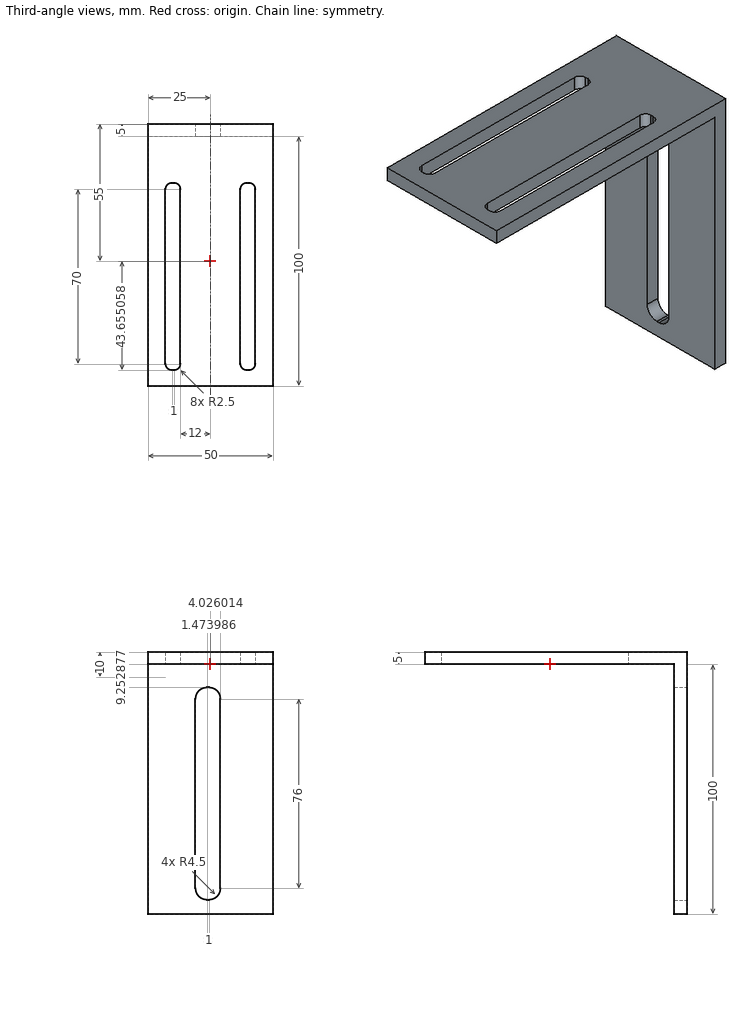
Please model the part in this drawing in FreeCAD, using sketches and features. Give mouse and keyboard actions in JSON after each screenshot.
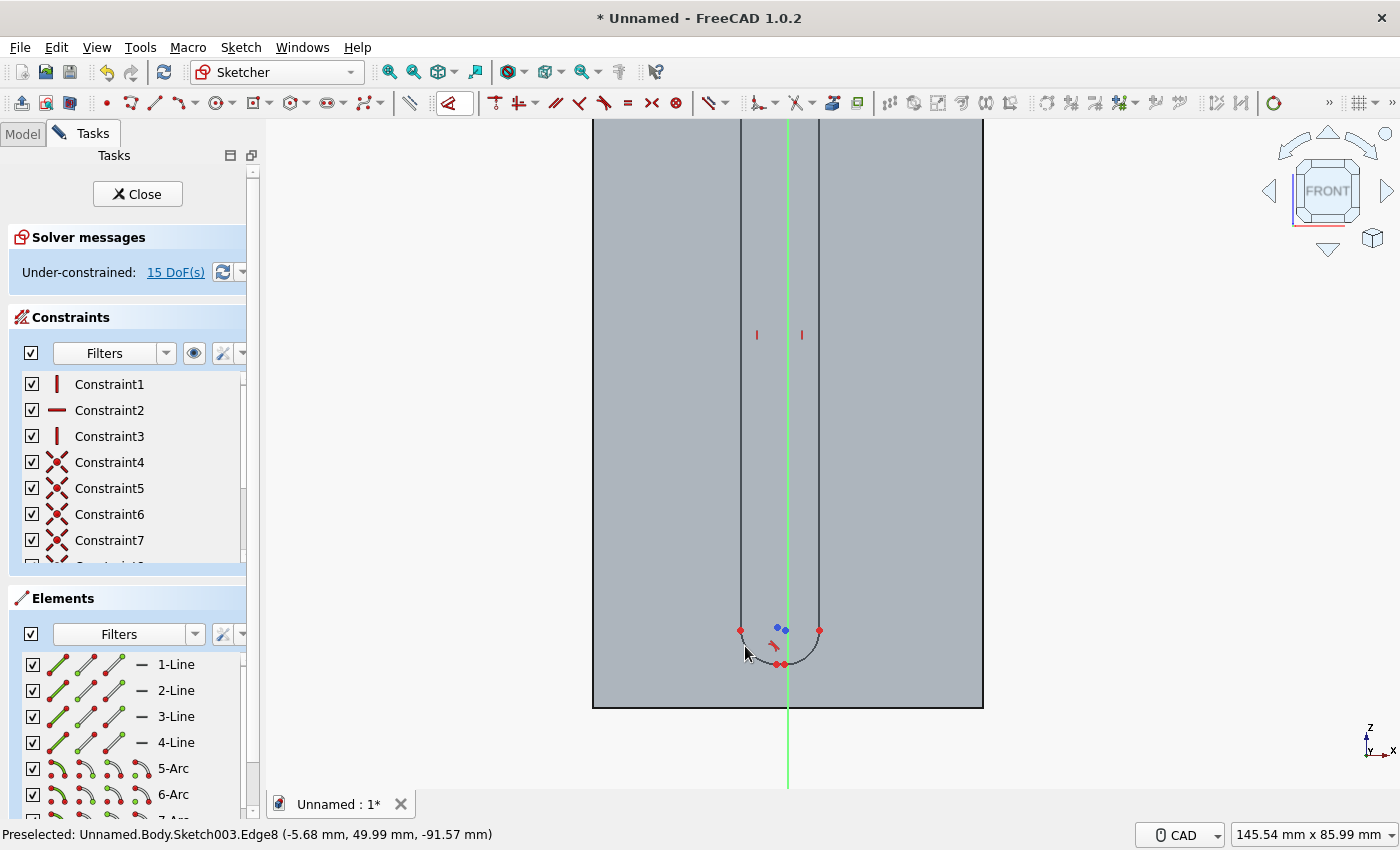
{"action": "left_click", "coordinate": [819, 453]}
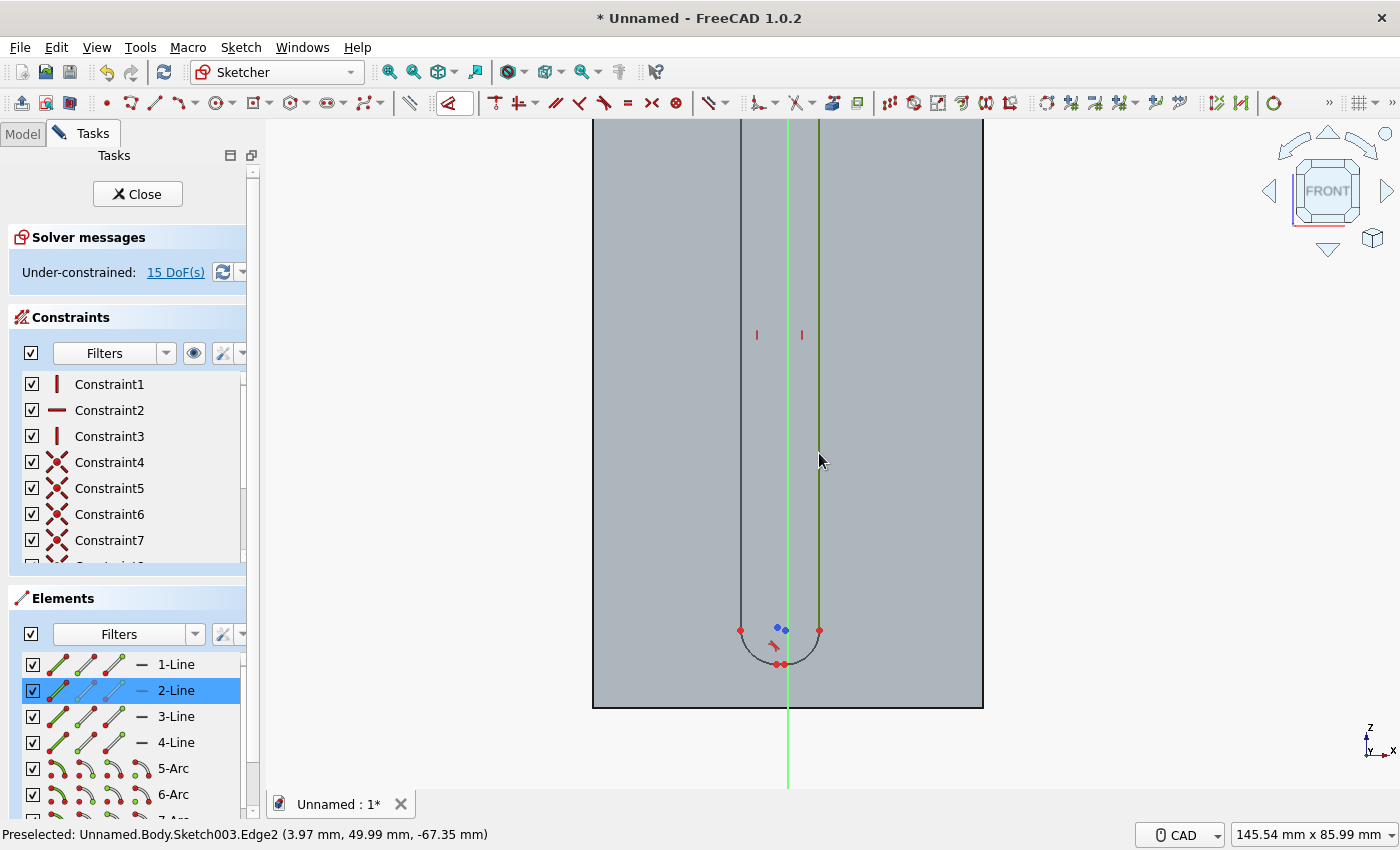
{"action": "left_click", "coordinate": [800, 661]}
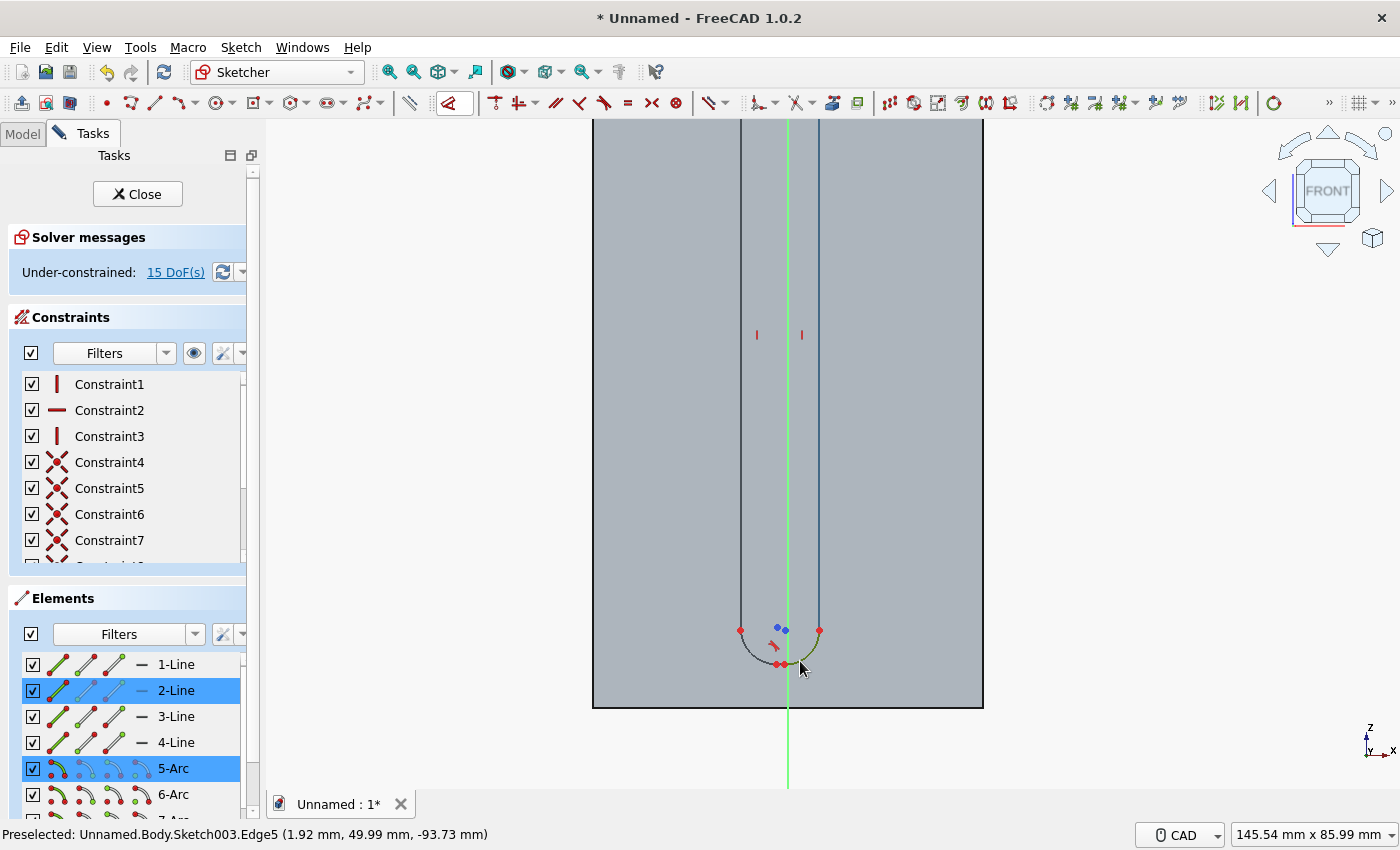
{"action": "left_click", "coordinate": [604, 104]}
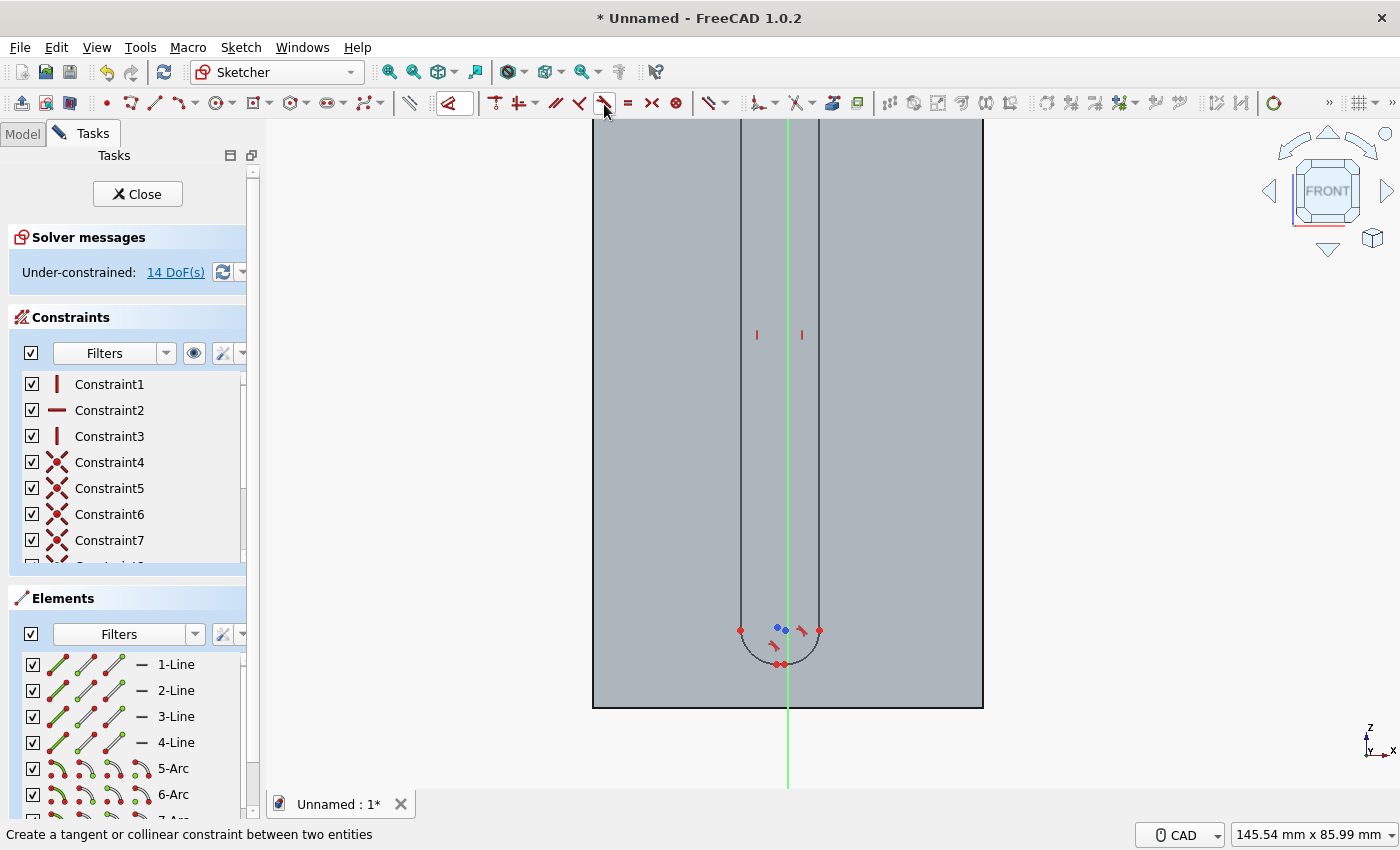
{"action": "left_click", "coordinate": [819, 453]}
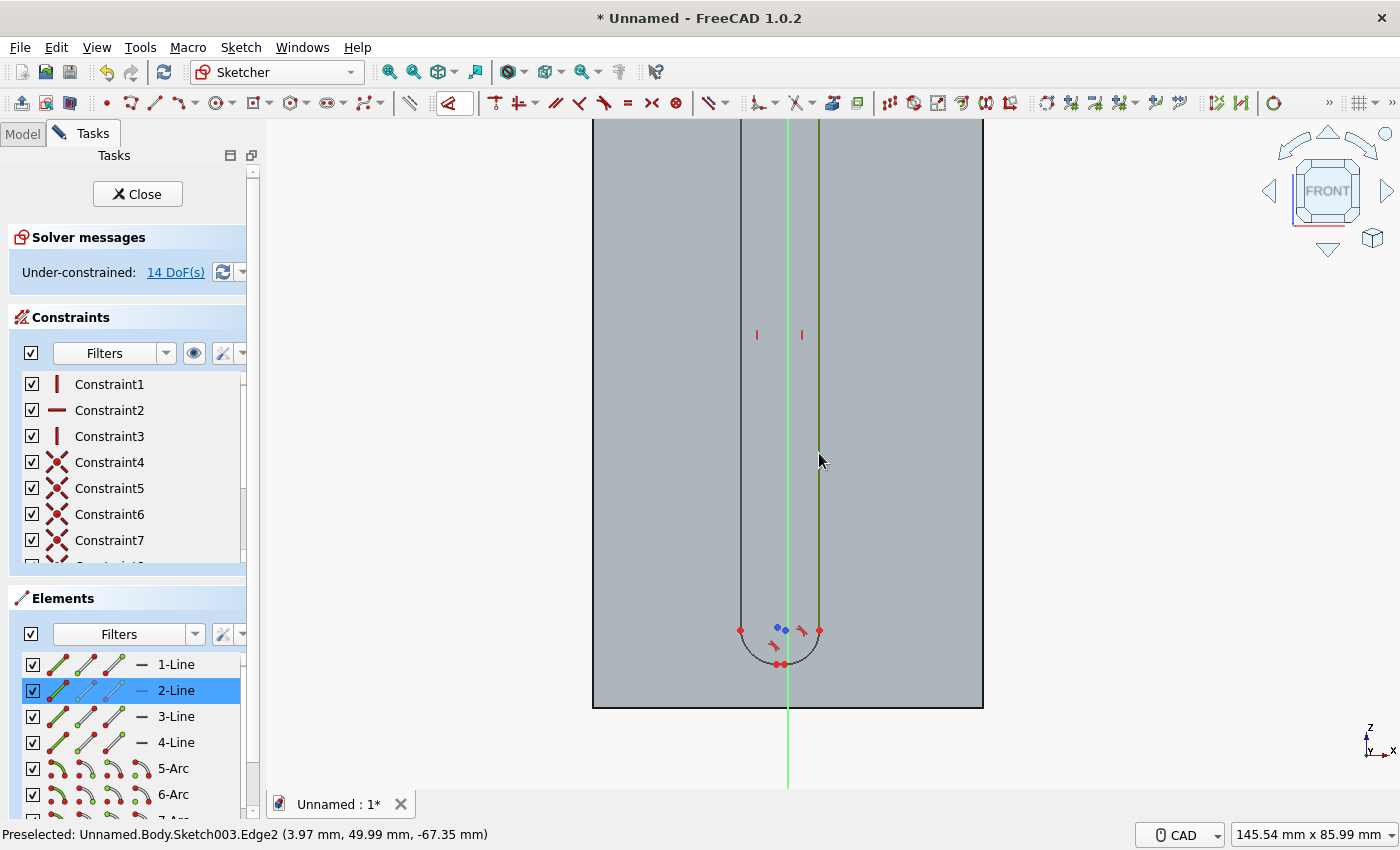
{"action": "scroll", "coordinate": [745, 646], "scroll_direction": "down", "scroll_amount": 3}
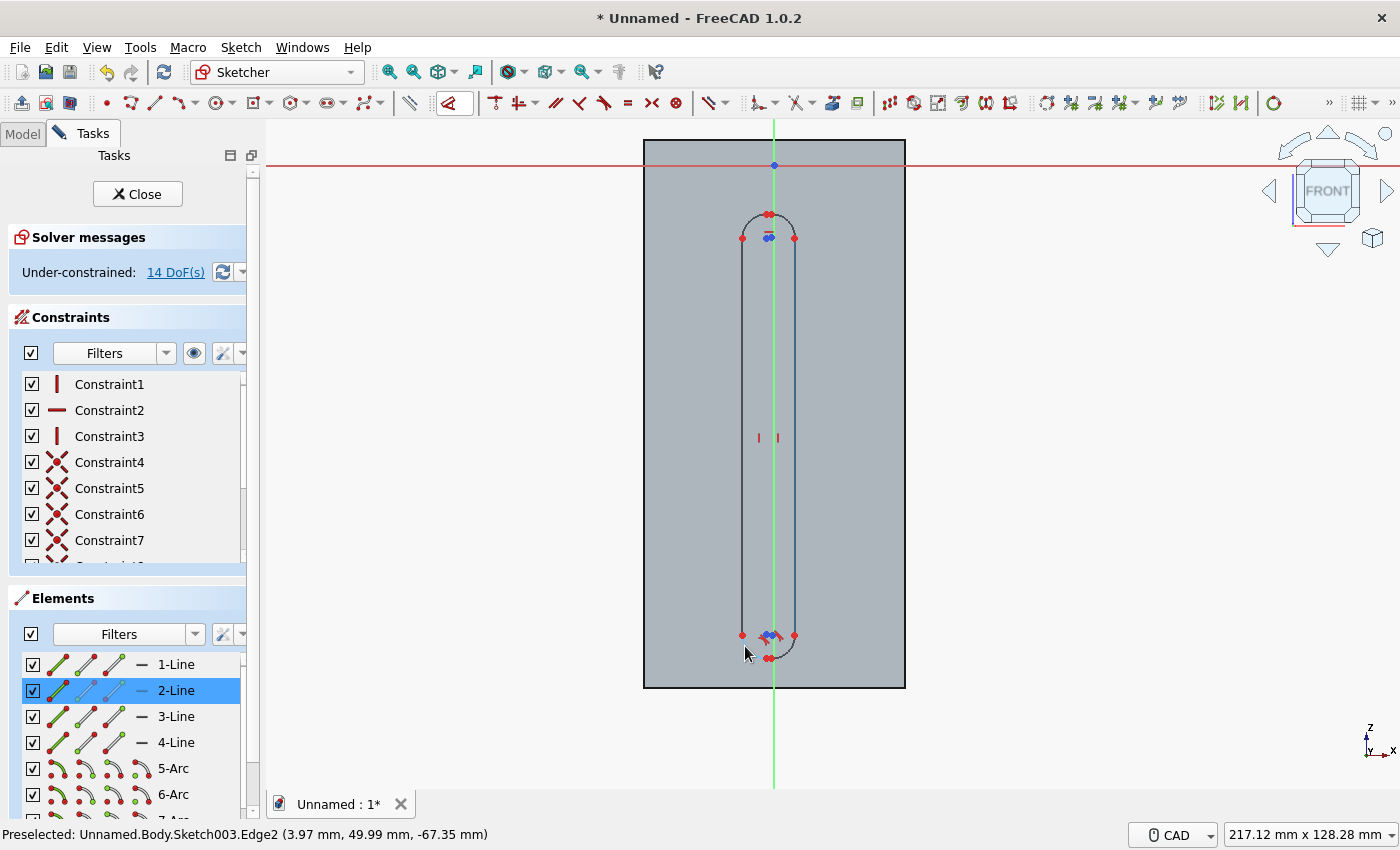
{"action": "scroll", "coordinate": [784, 304], "scroll_direction": "up", "scroll_amount": 3}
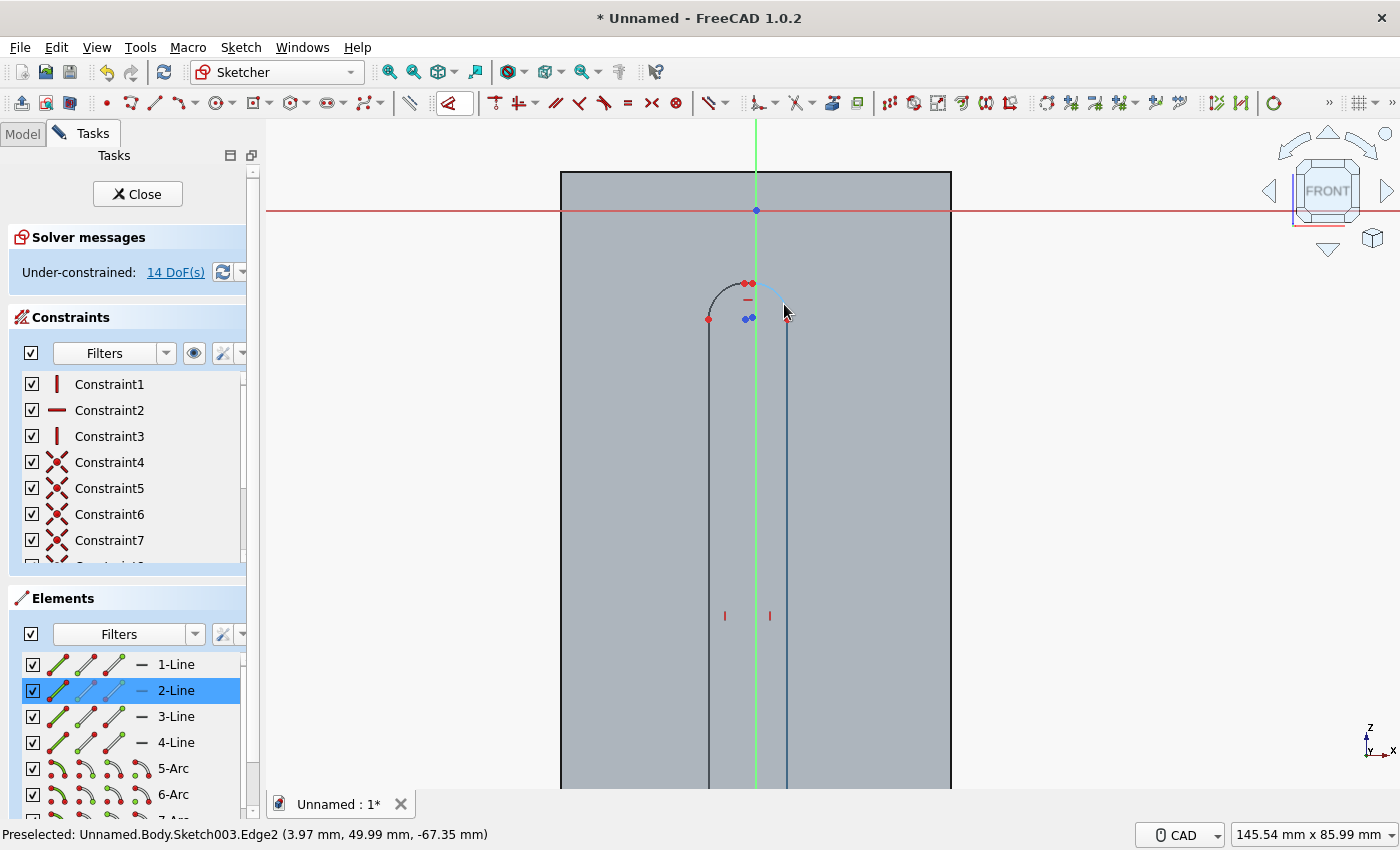
{"action": "left_click", "coordinate": [784, 303]}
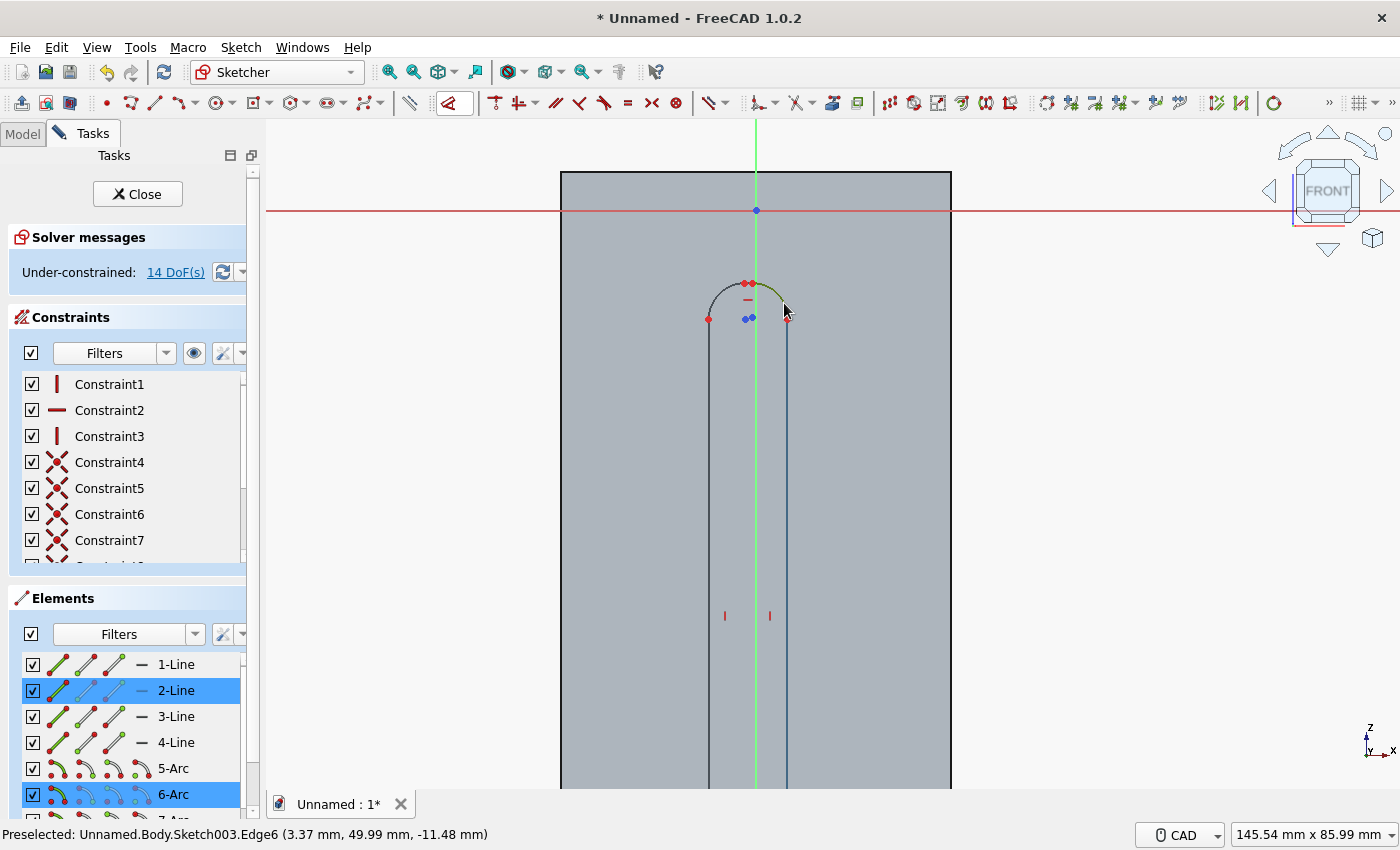
{"action": "key", "text": "t"}